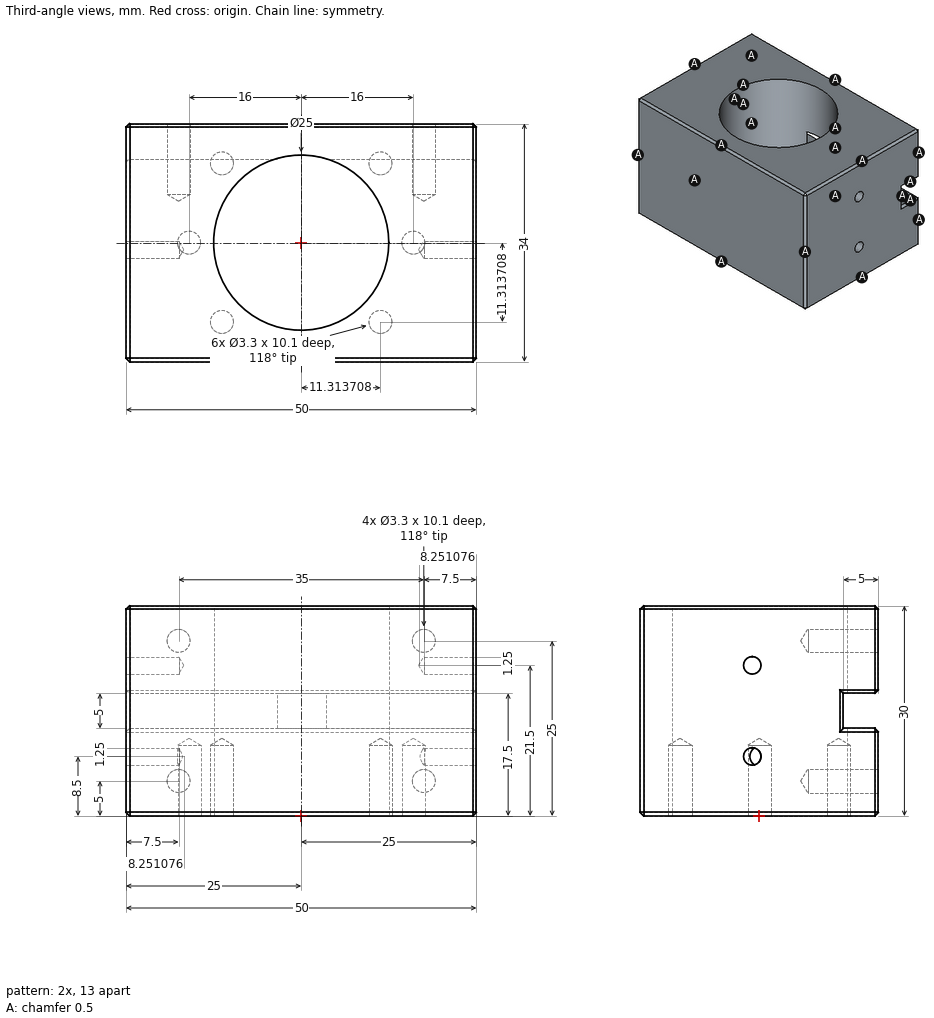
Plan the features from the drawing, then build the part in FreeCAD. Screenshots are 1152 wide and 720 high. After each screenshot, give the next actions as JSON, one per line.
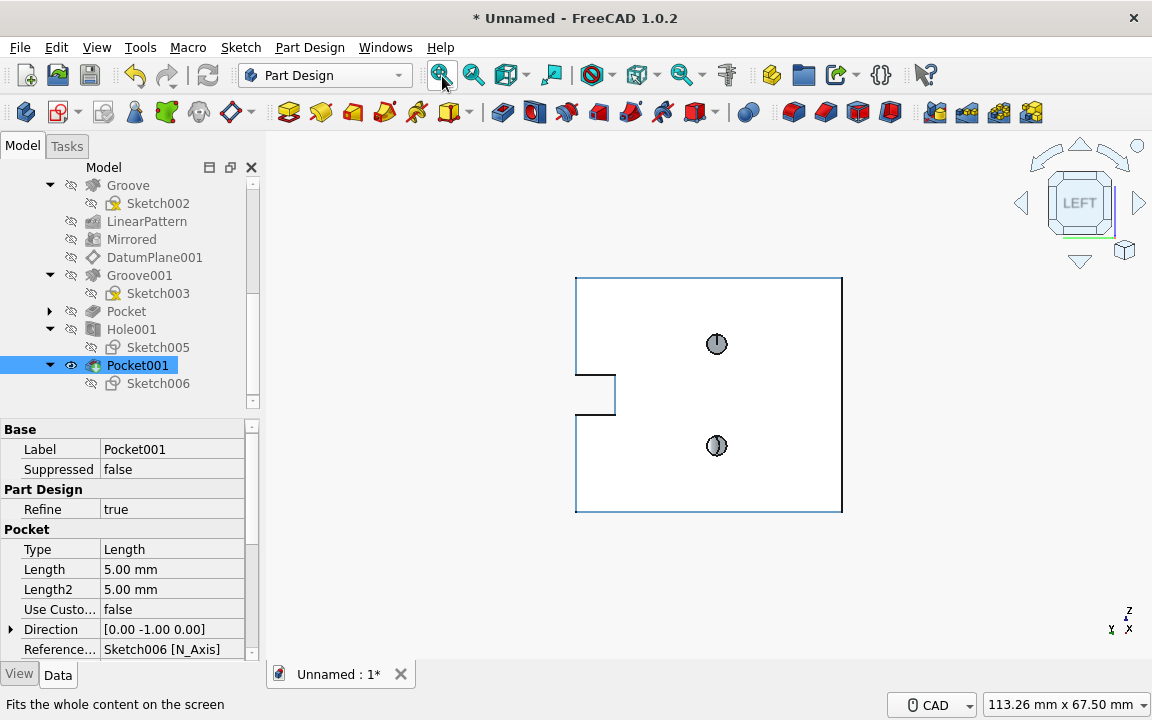
{"action": "left_click", "coordinate": [442, 76]}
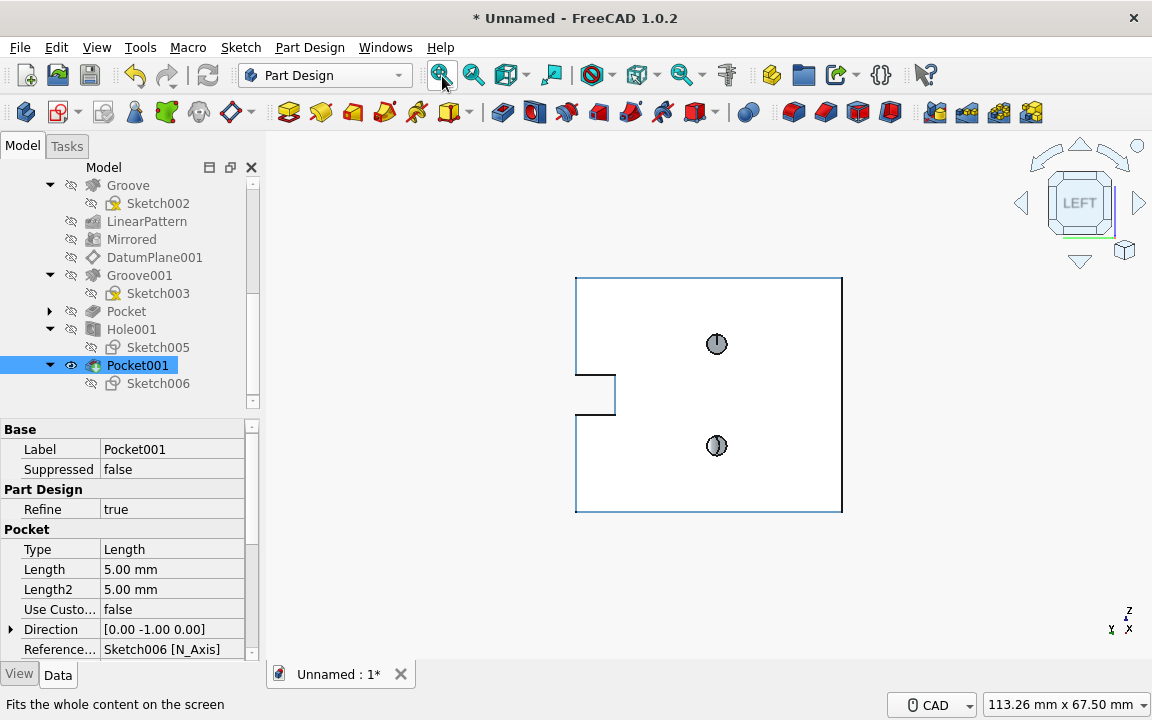
{"action": "left_click", "coordinate": [596, 414], "text": "ctrl"}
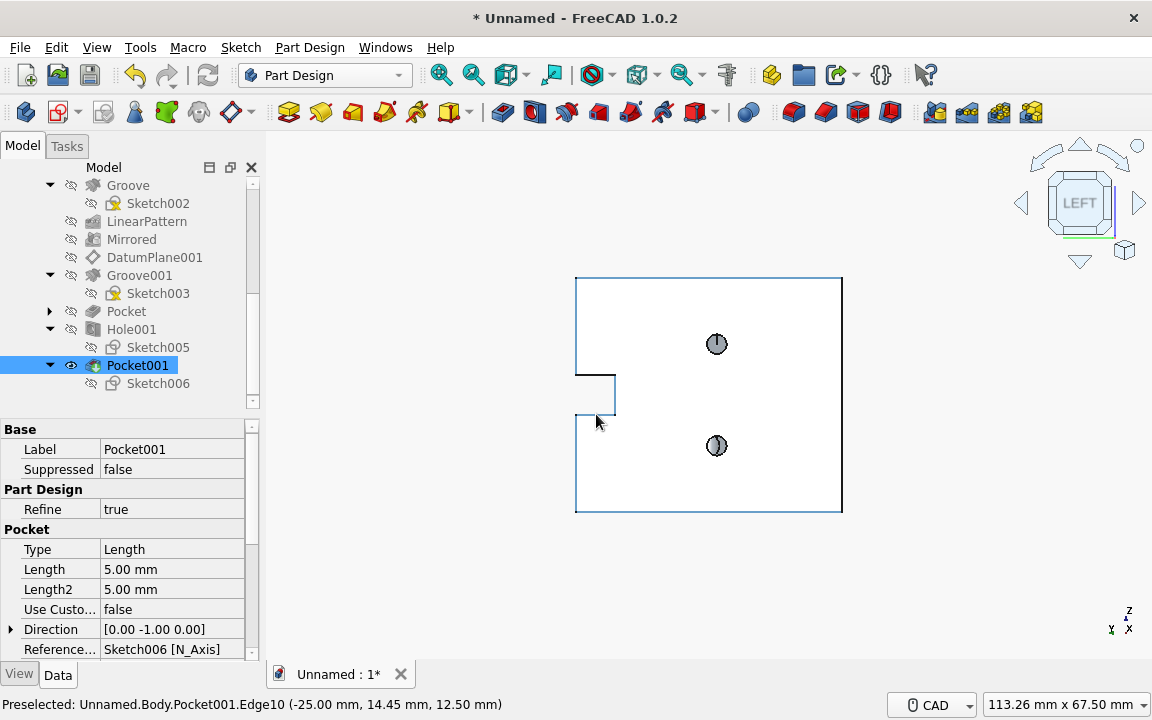
{"action": "left_click", "coordinate": [596, 374], "text": "ctrl"}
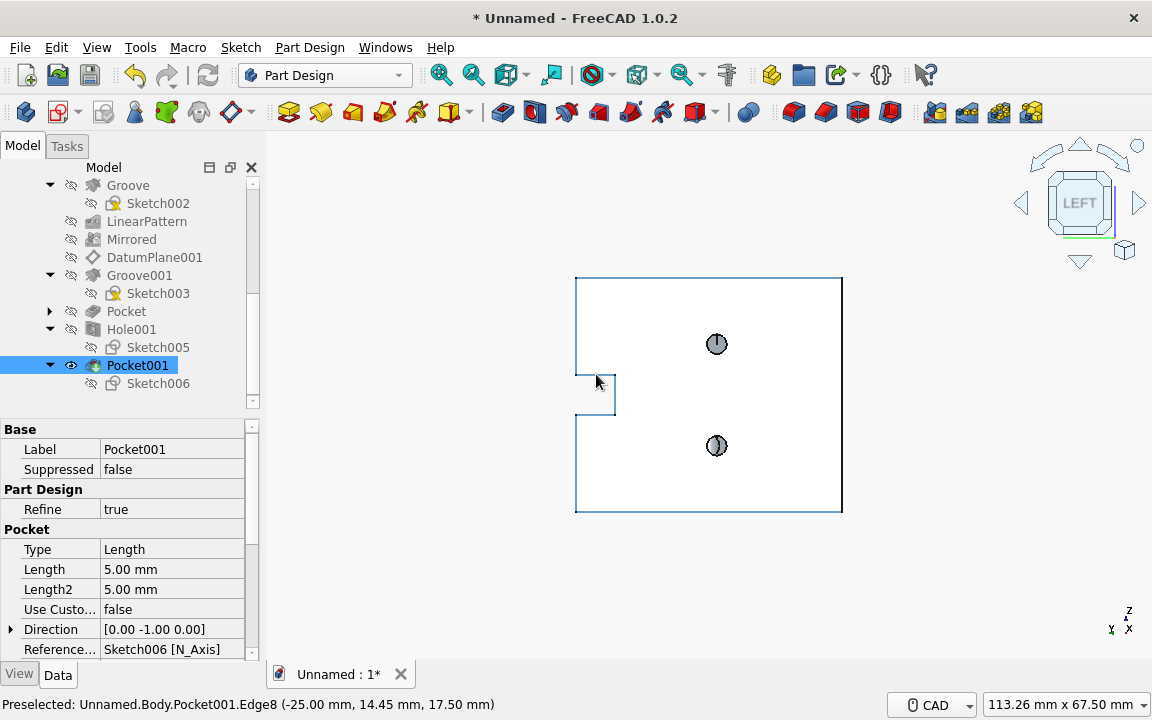
{"action": "left_click", "coordinate": [826, 112]}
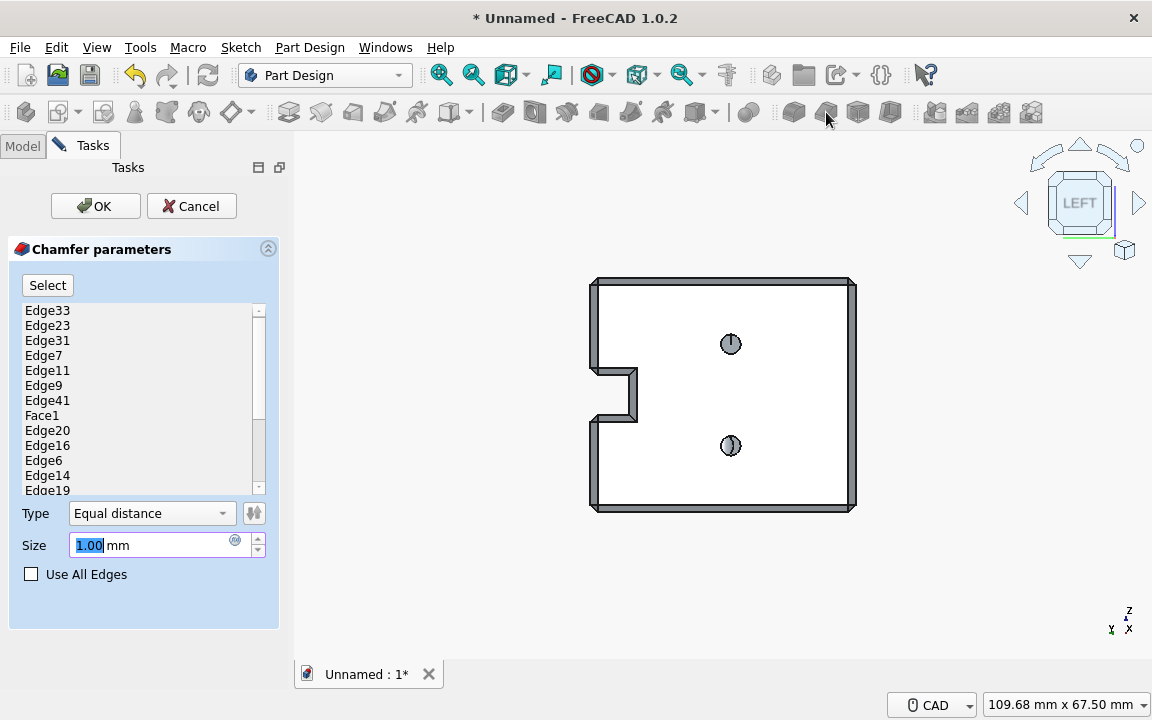
{"action": "type", "text": "0.5"}
{"action": "key", "text": "Tab"}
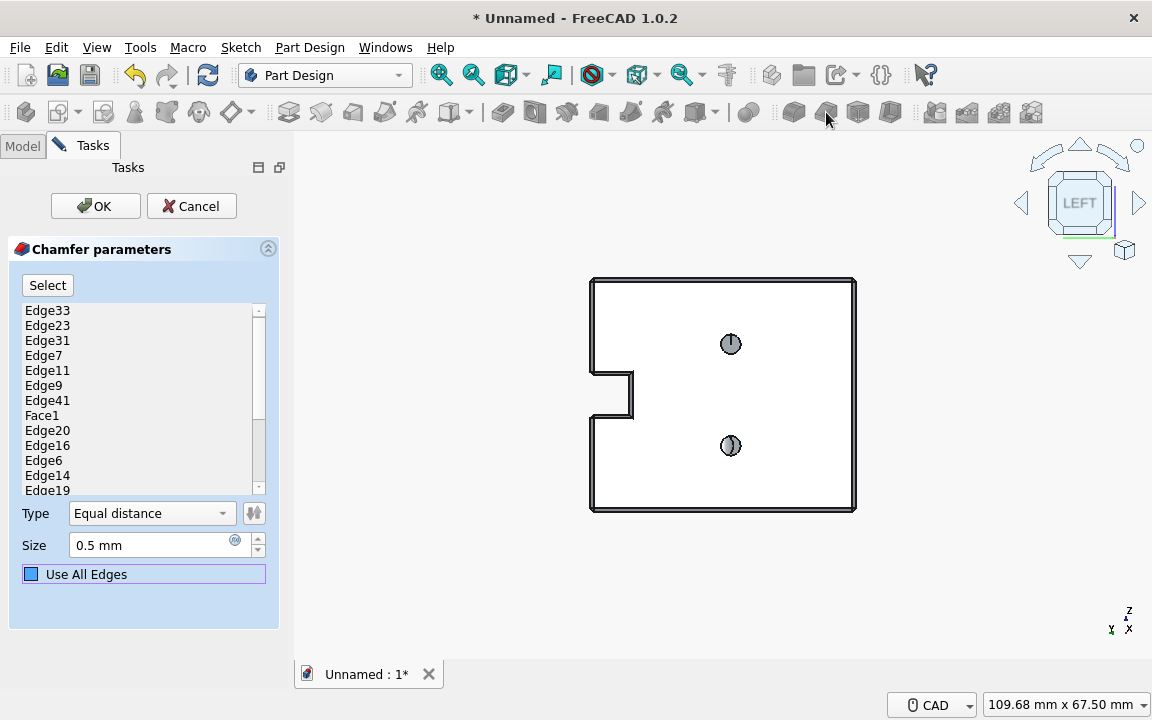
{"action": "left_click", "coordinate": [96, 206]}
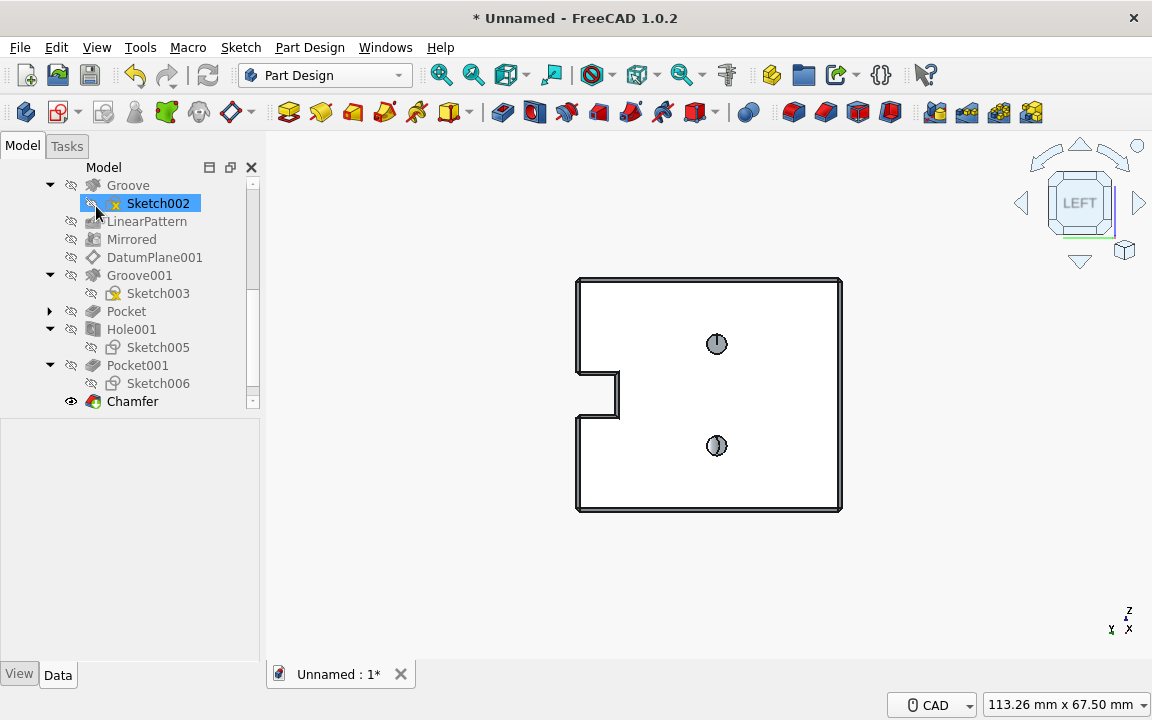
{"action": "key", "text": "0"}